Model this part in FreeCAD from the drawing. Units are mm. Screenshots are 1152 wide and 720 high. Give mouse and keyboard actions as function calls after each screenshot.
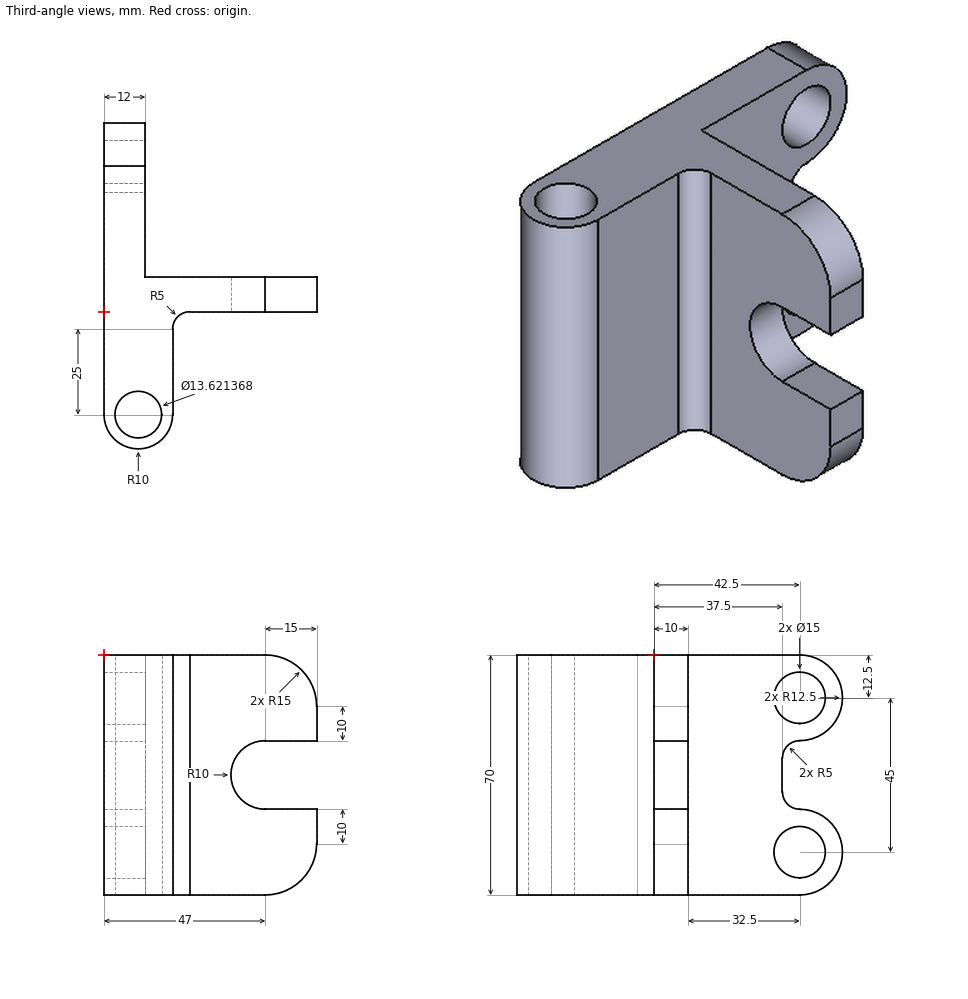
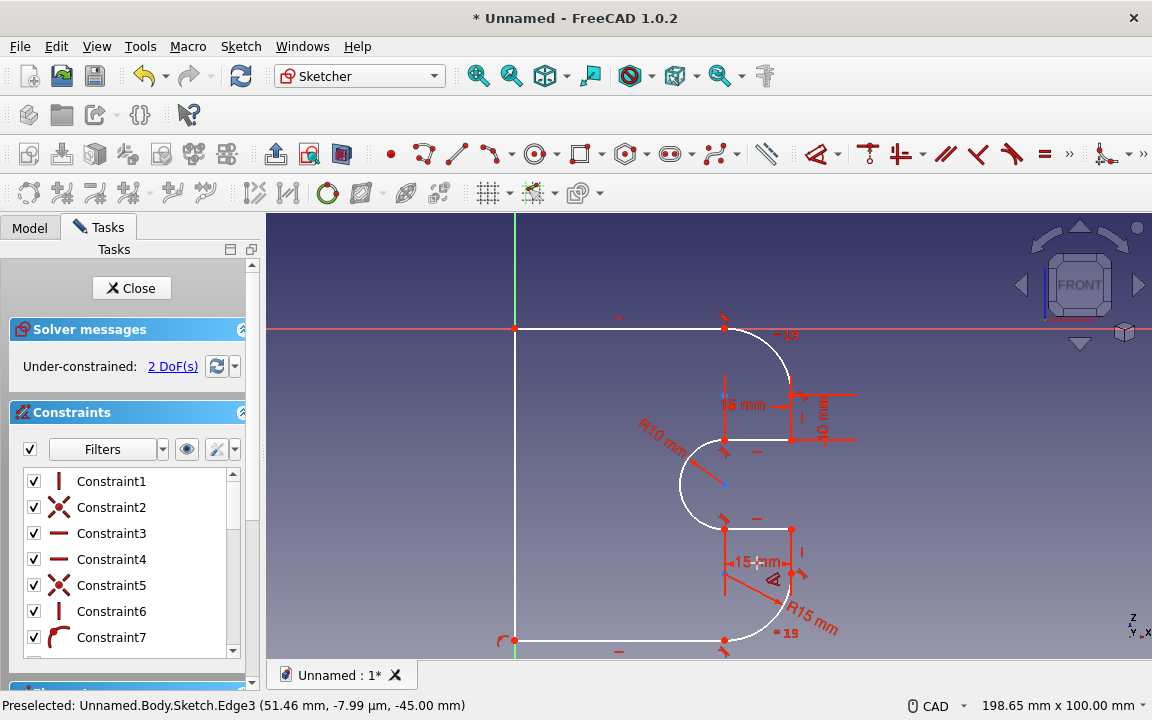
click(791, 543)
click(825, 541)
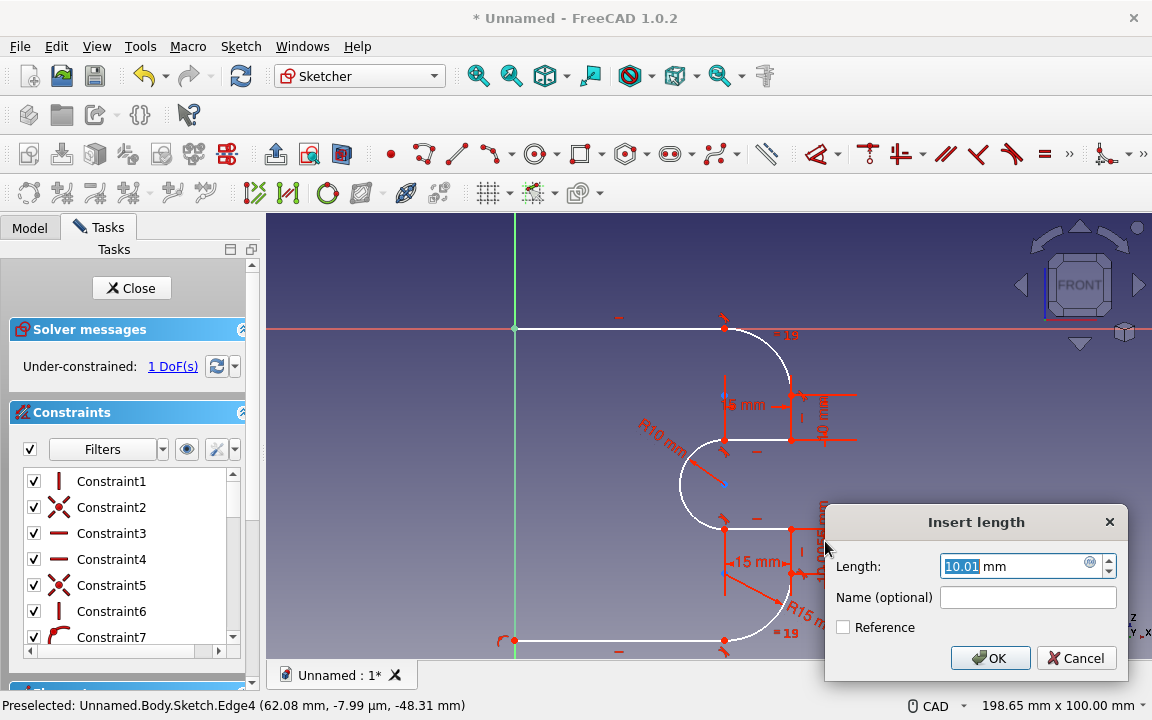
text(10)
key(Return)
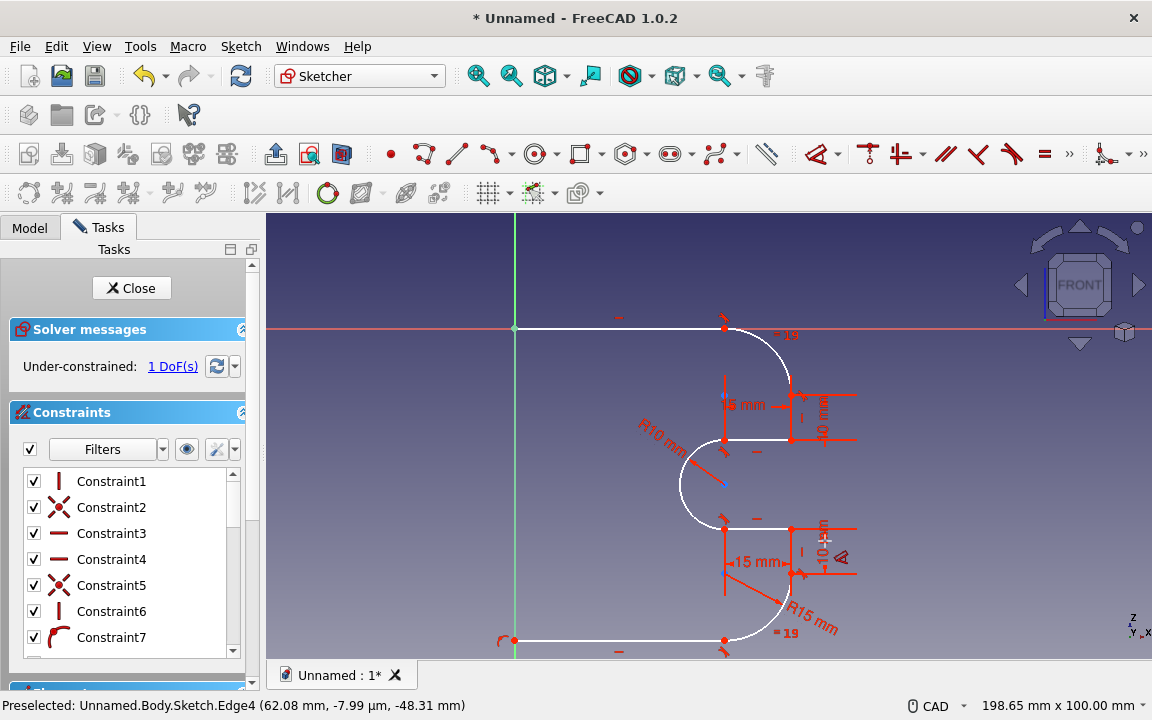
scroll(585, 241, down, 1)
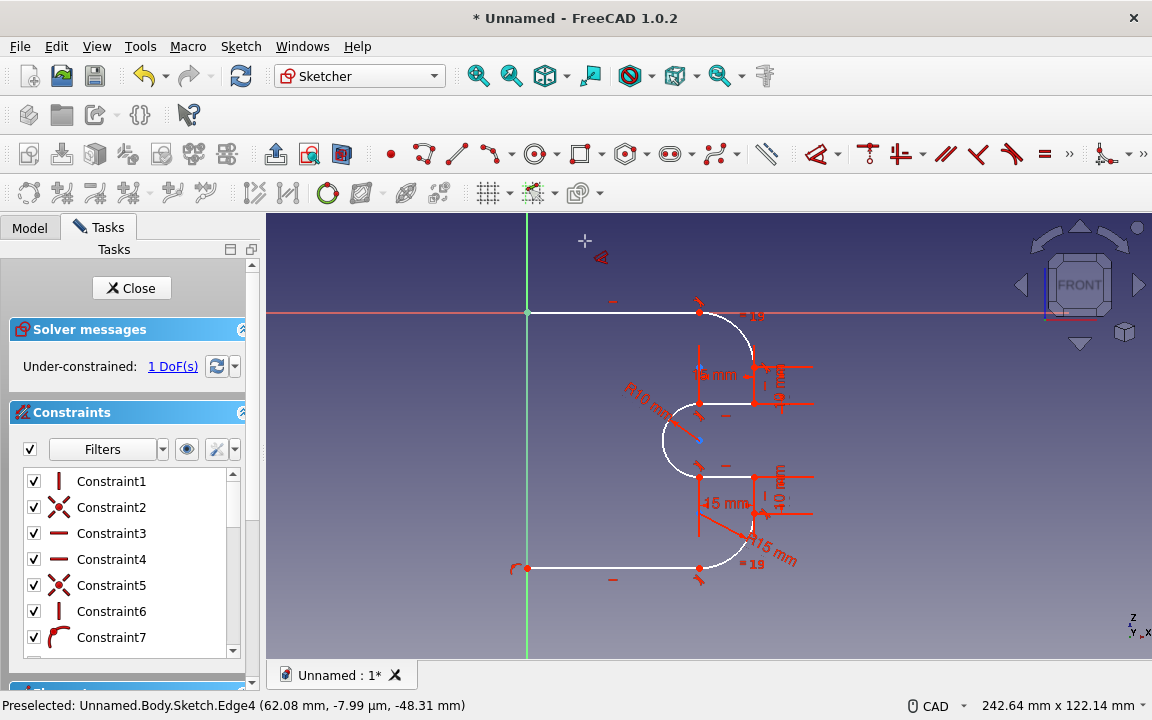
click(648, 568)
click(613, 602)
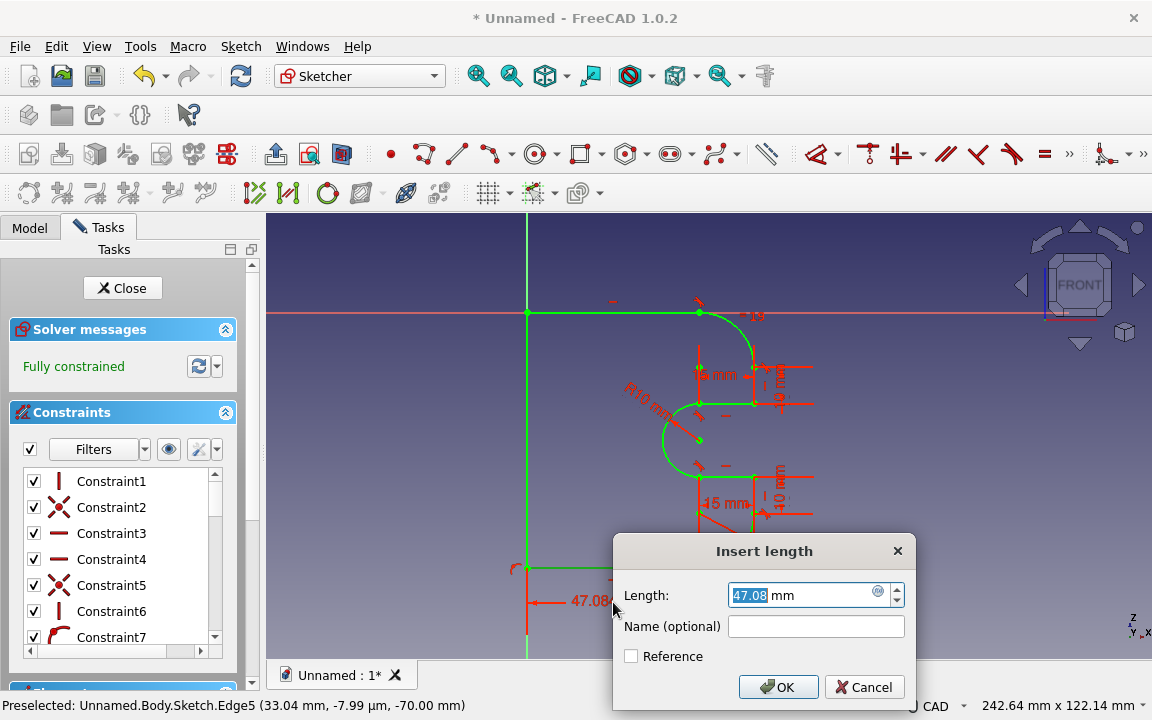
text(47)
key(Return)
key(Escape)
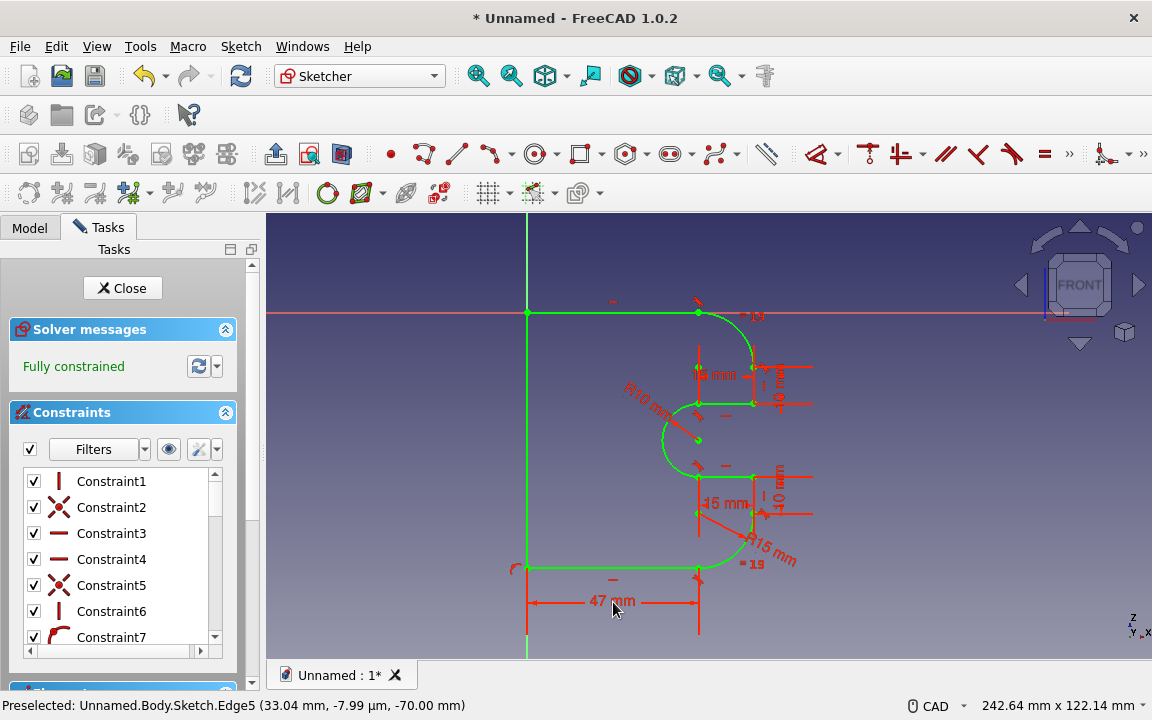
click(123, 288)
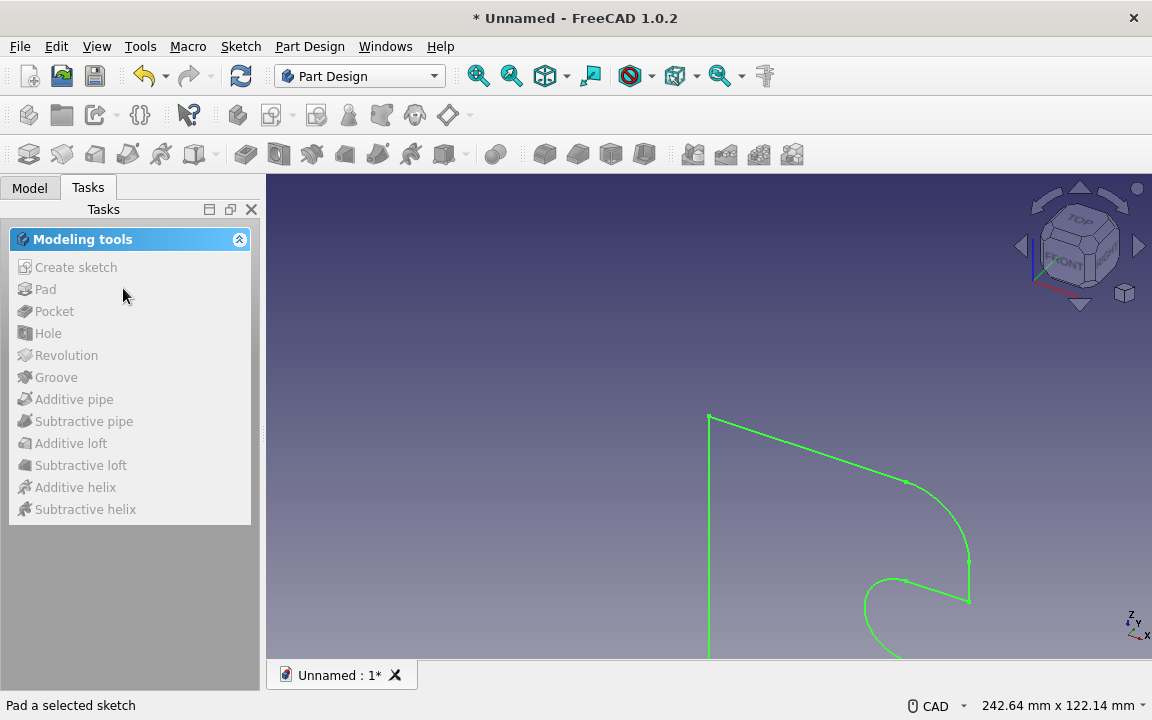
click(29, 154)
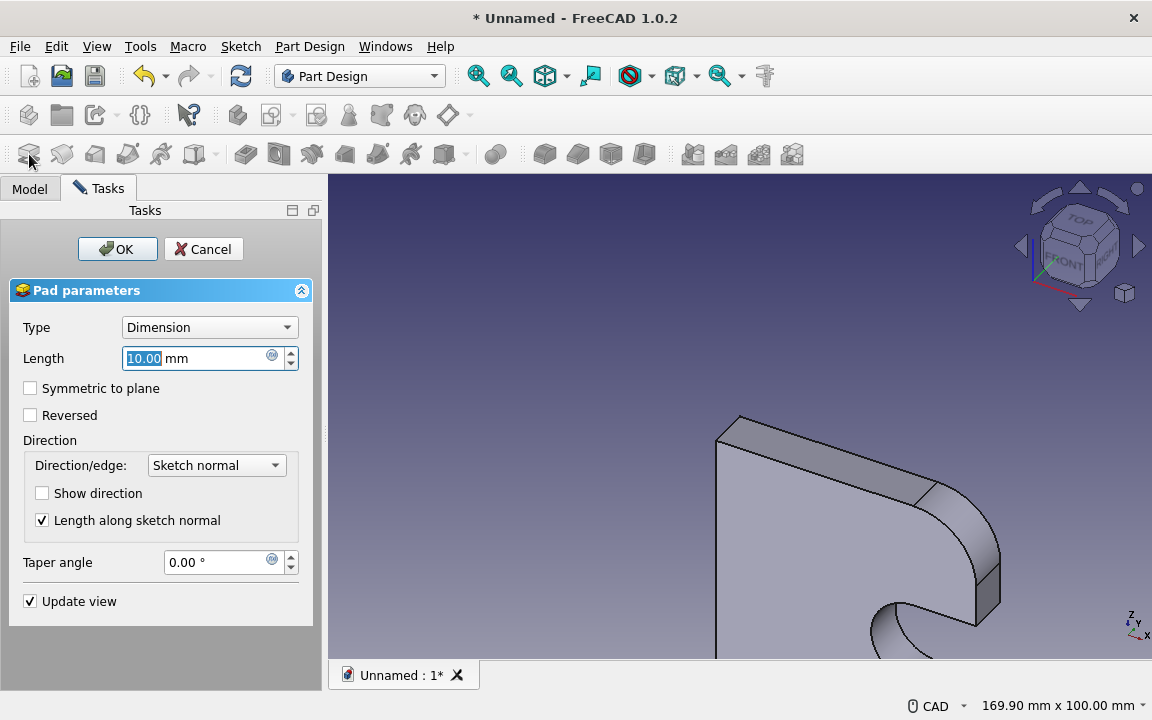
text(10)
key(Tab)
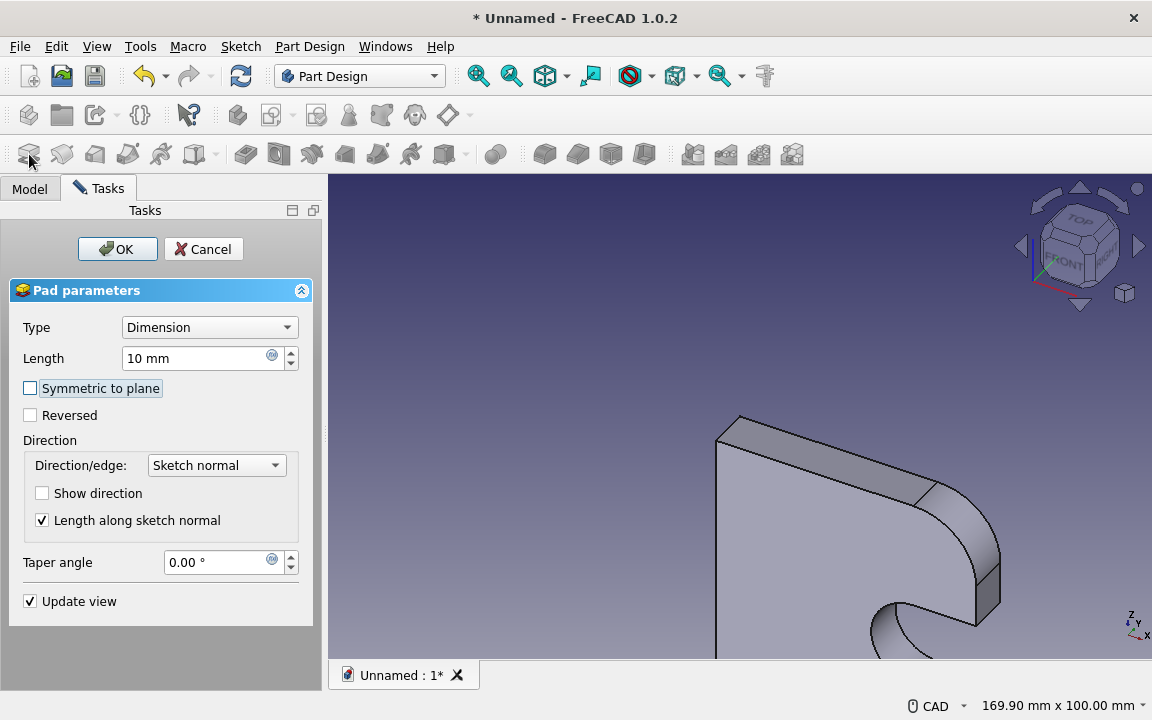
click(31, 415)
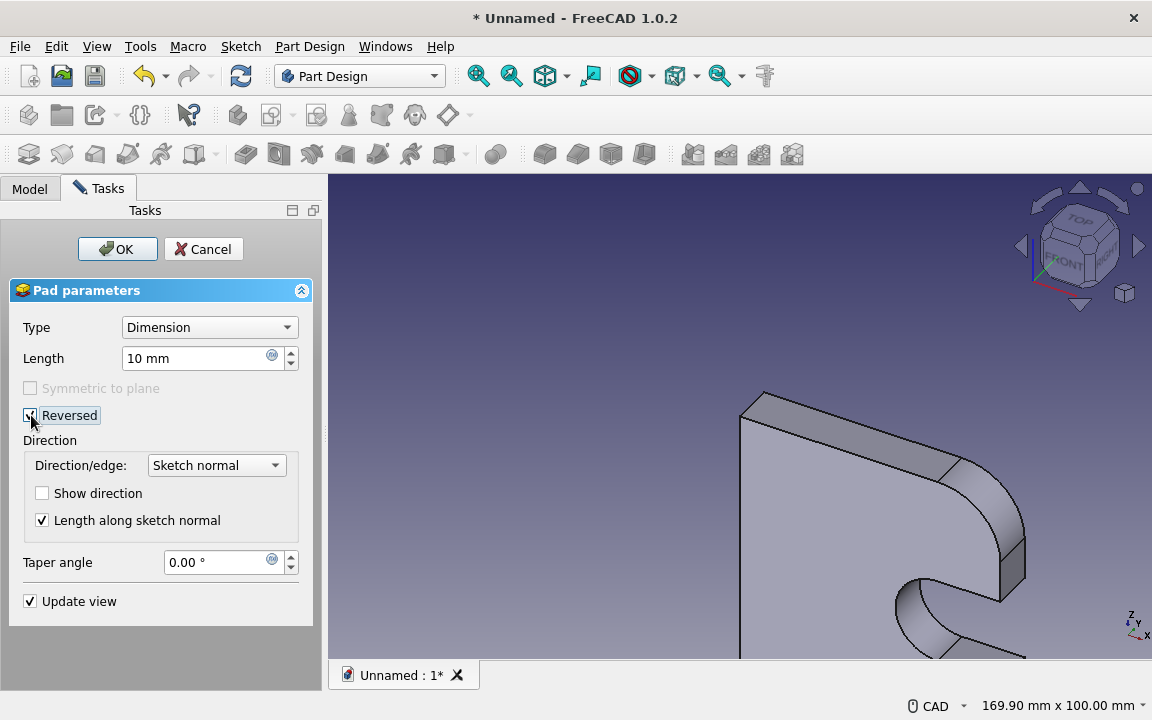
click(118, 249)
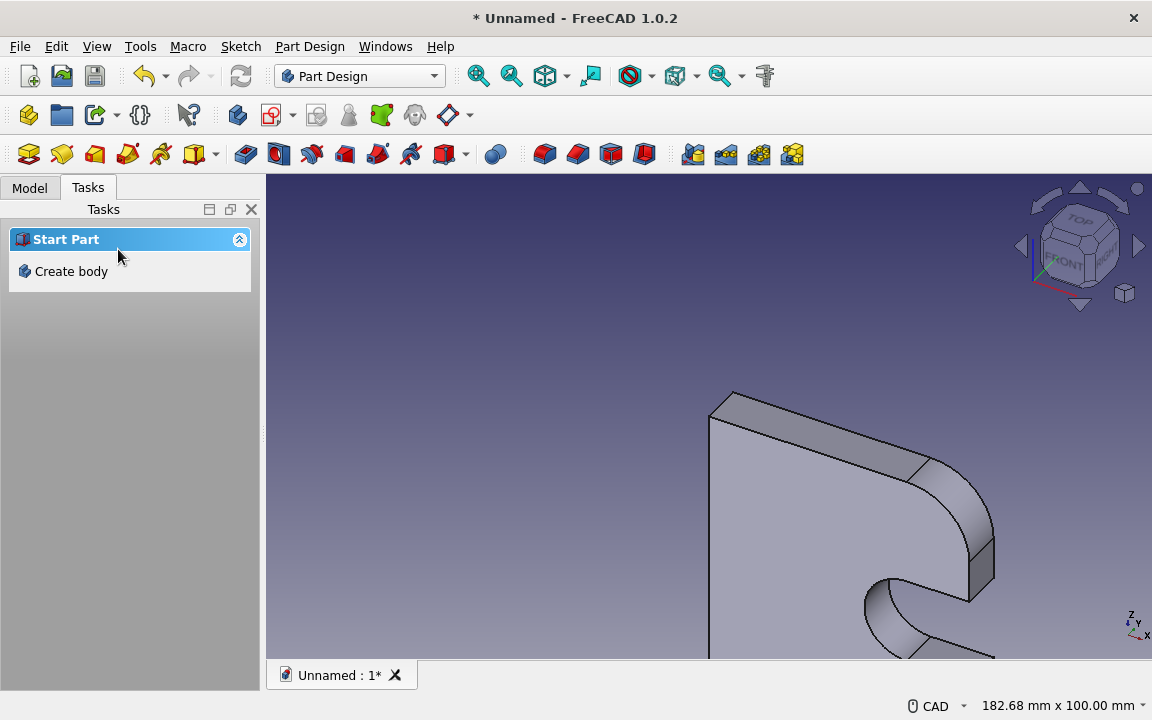
click(479, 76)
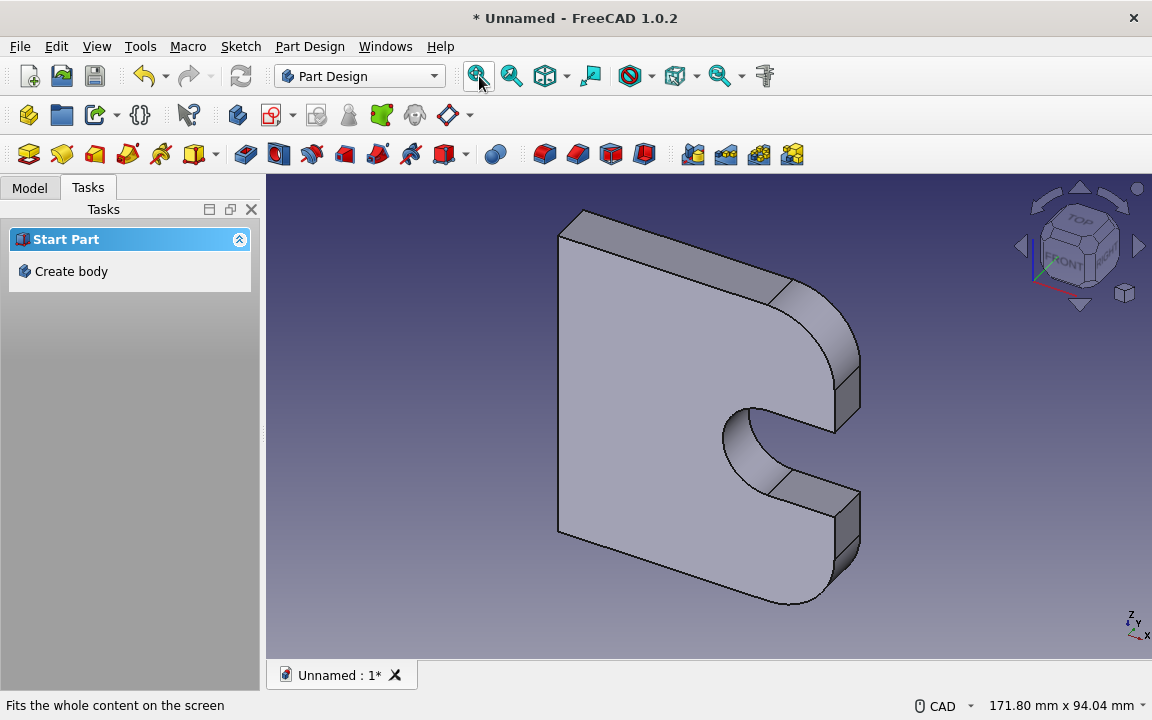
click(270, 116)